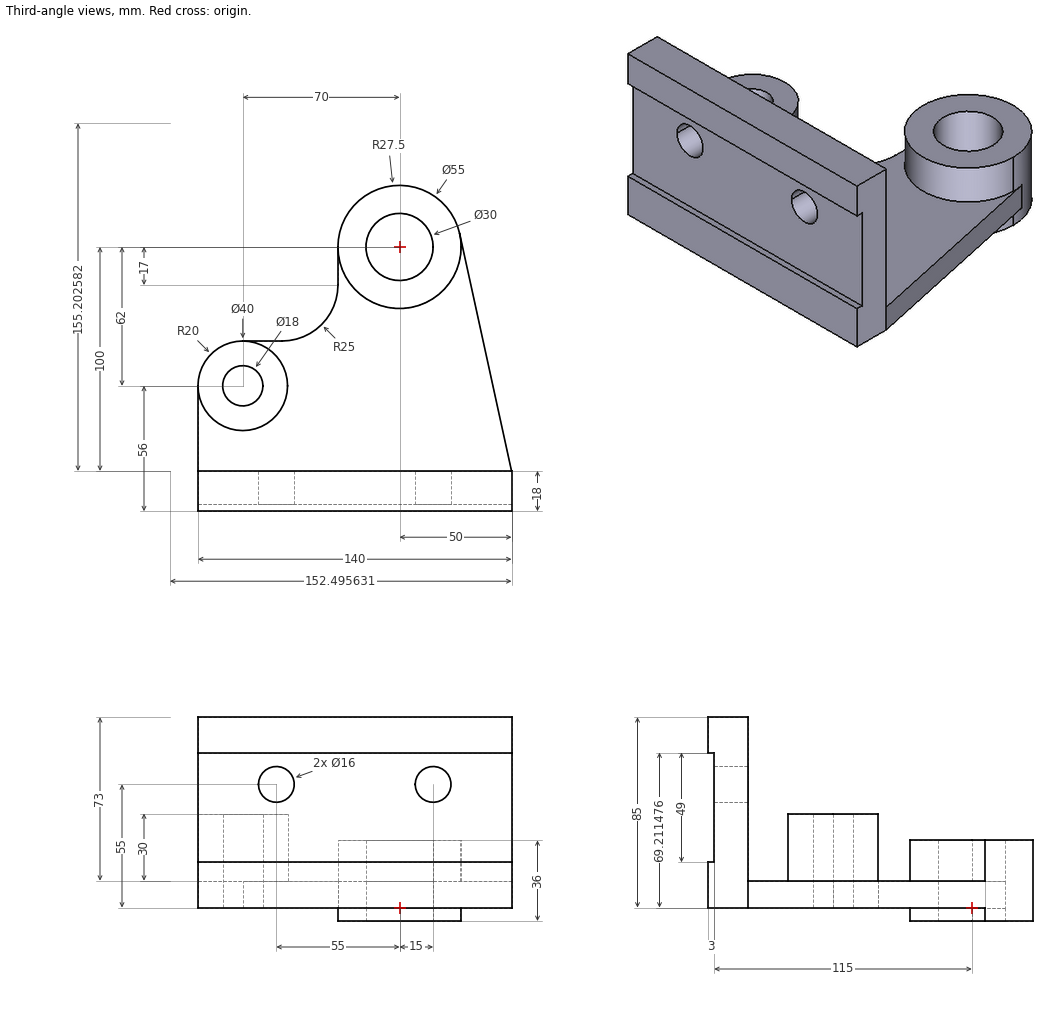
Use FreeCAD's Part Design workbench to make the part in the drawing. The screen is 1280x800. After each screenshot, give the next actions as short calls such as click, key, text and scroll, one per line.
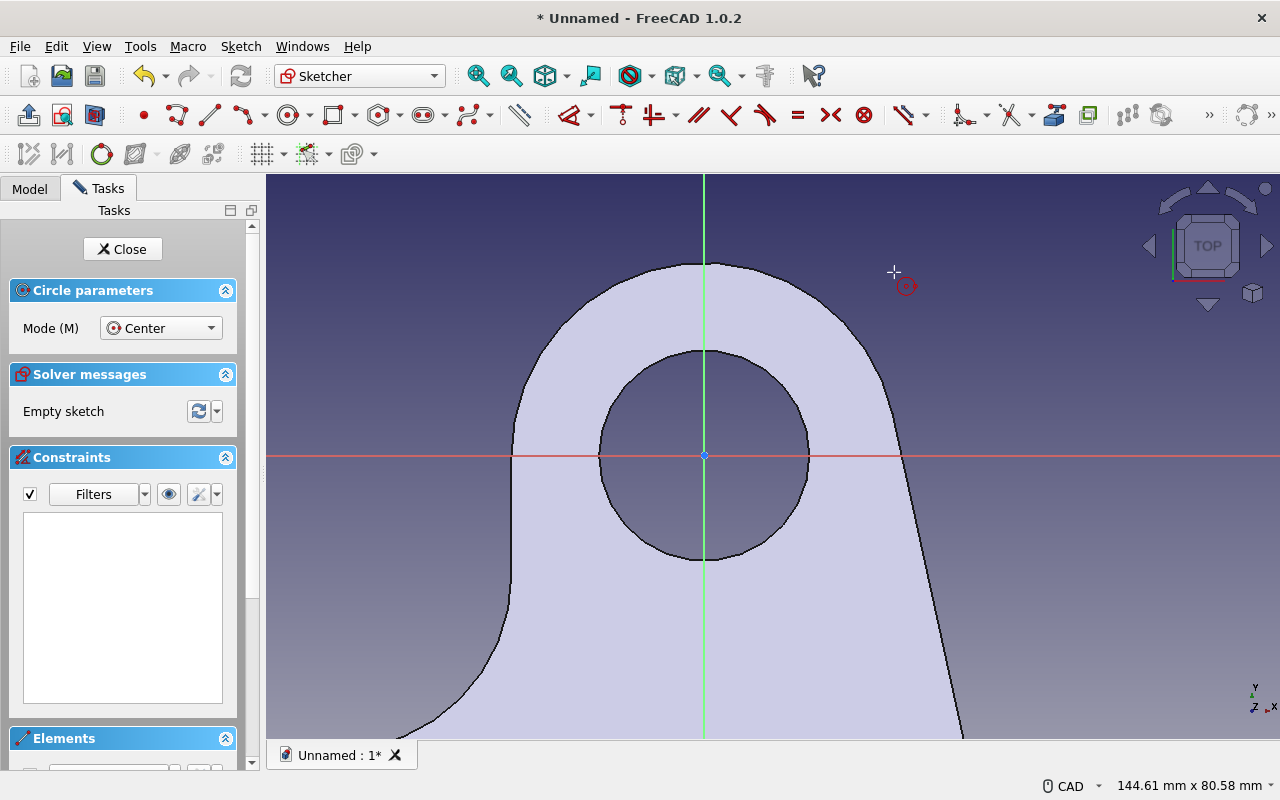
click(704, 456)
click(841, 319)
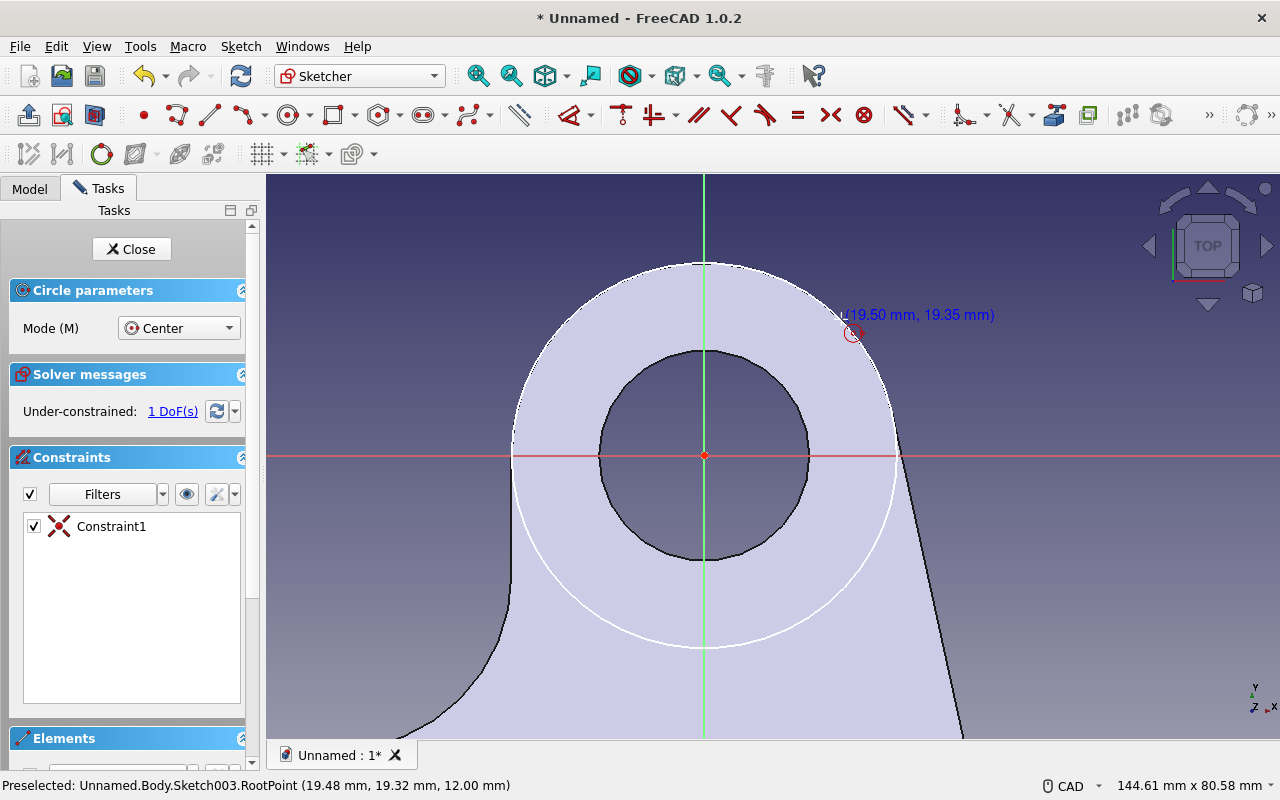
click(704, 456)
click(779, 381)
key(Escape)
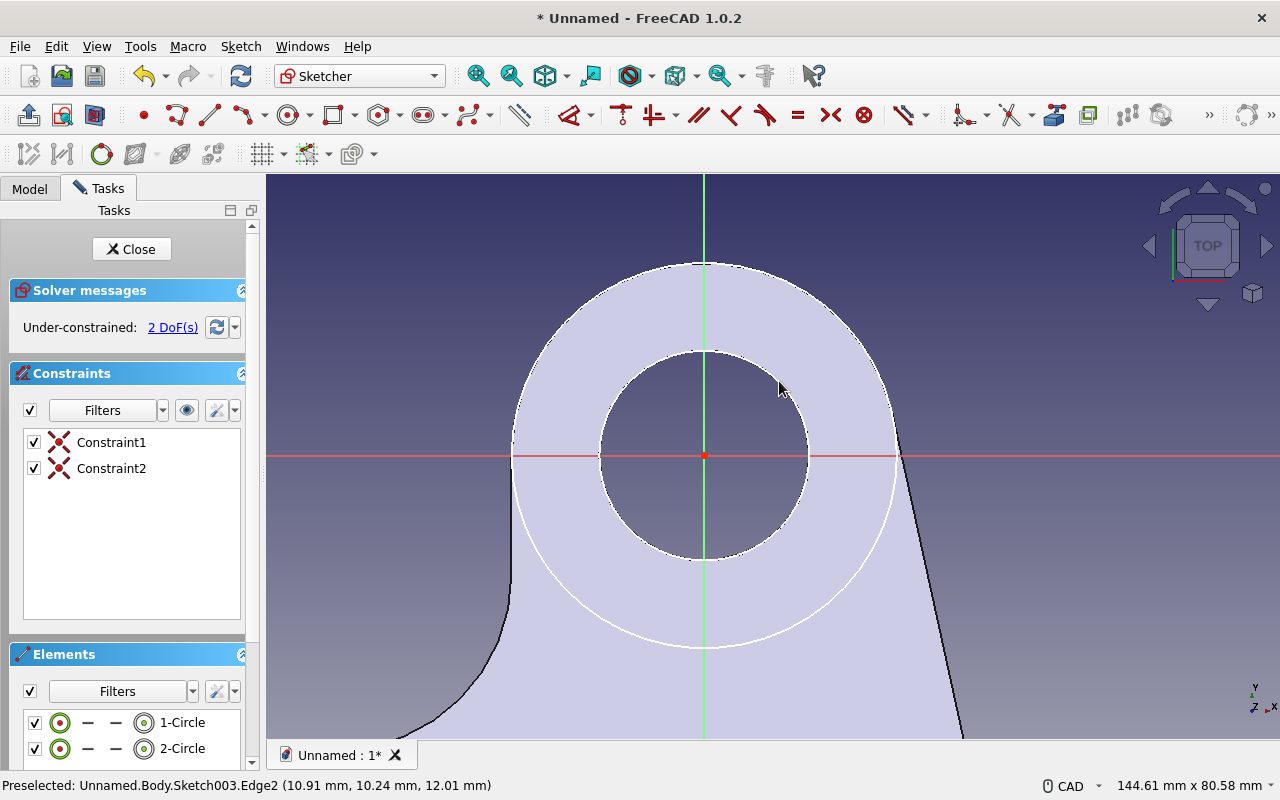
click(568, 116)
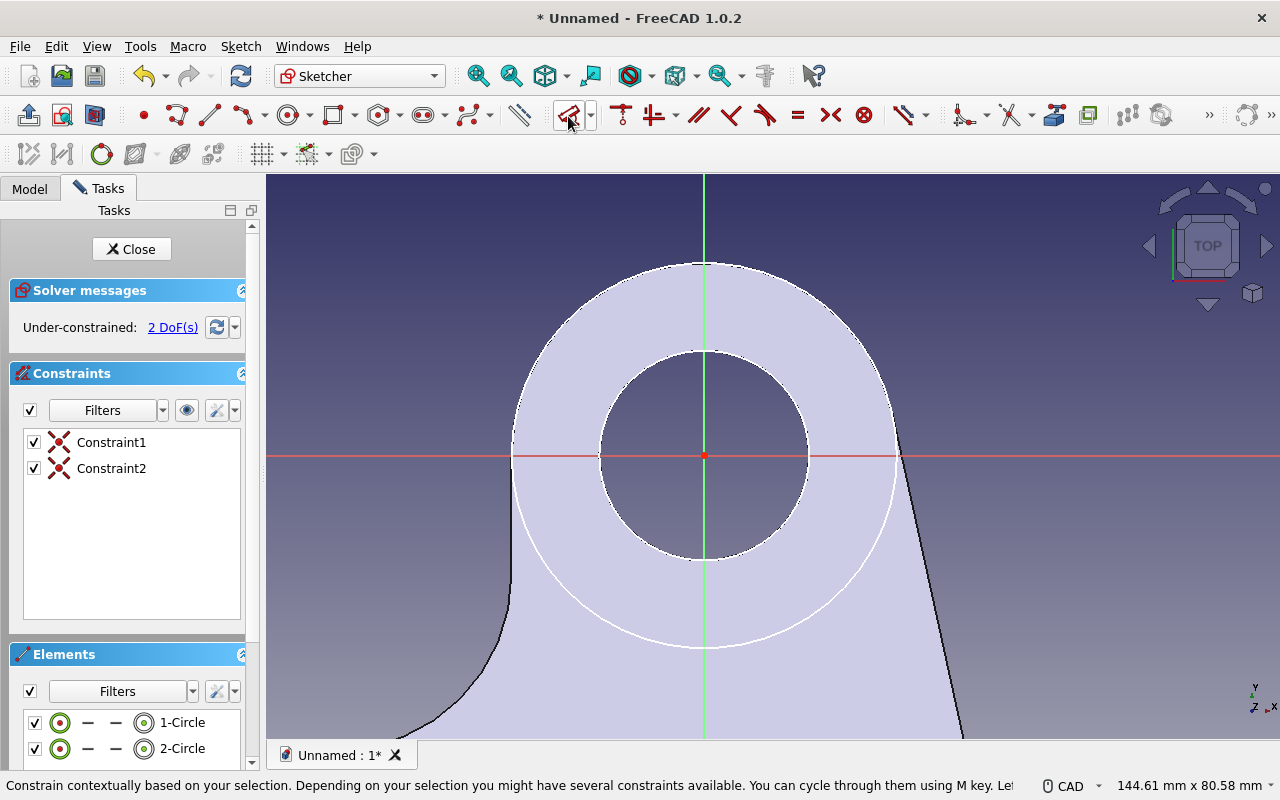
click(840, 319)
click(863, 296)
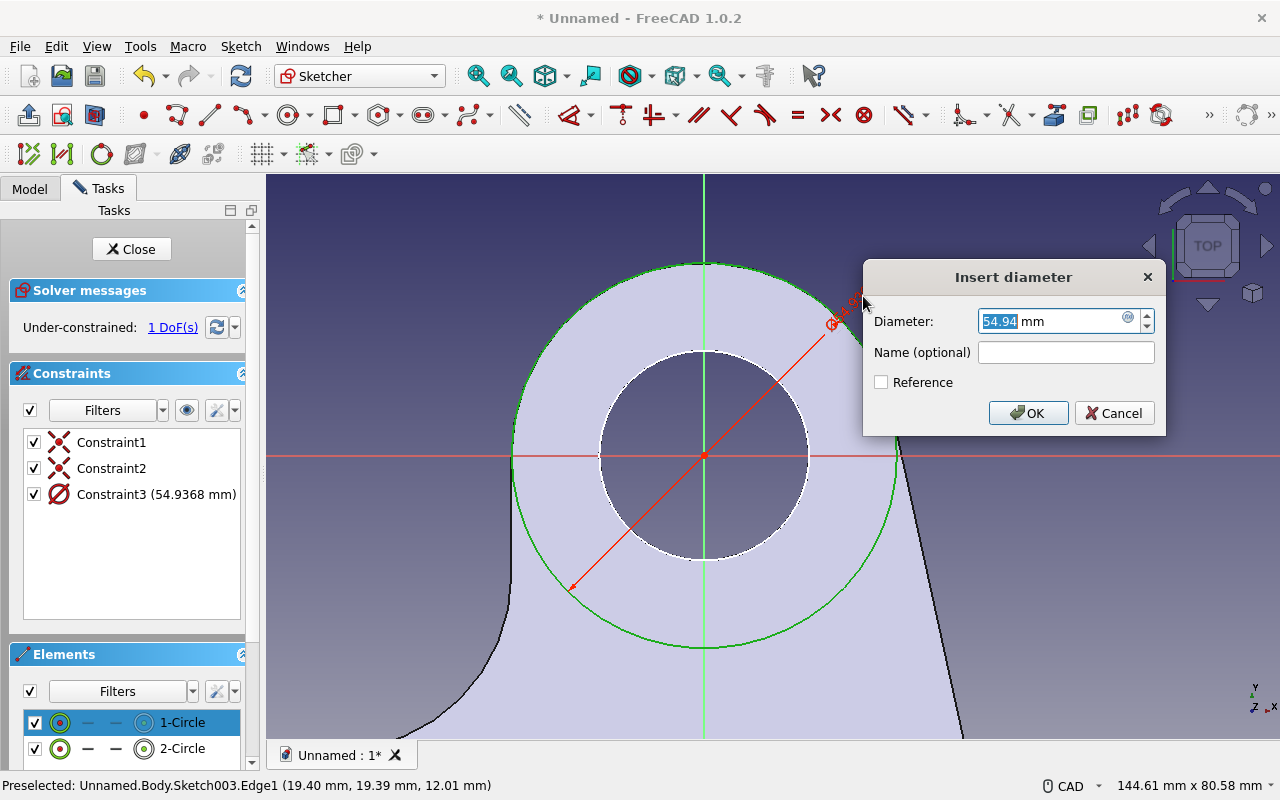
text(55)
key(Return)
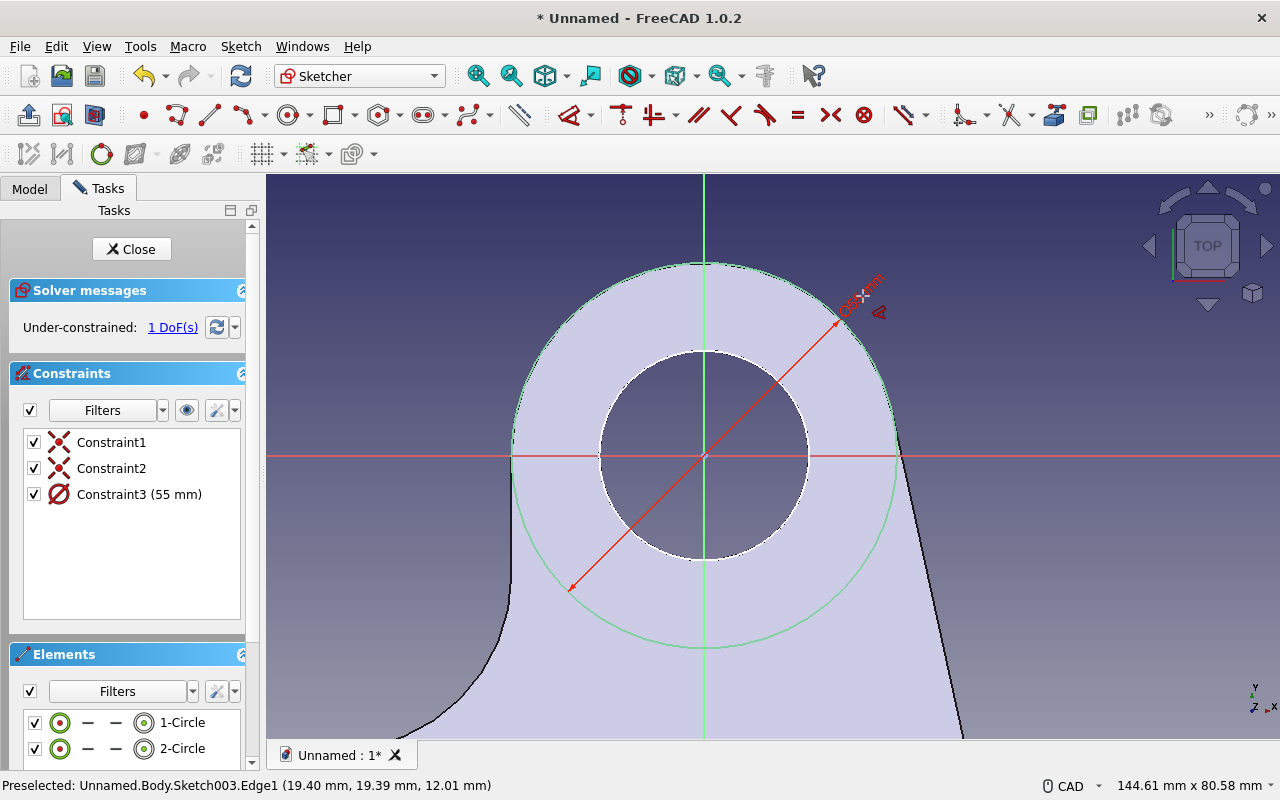
click(778, 381)
click(800, 358)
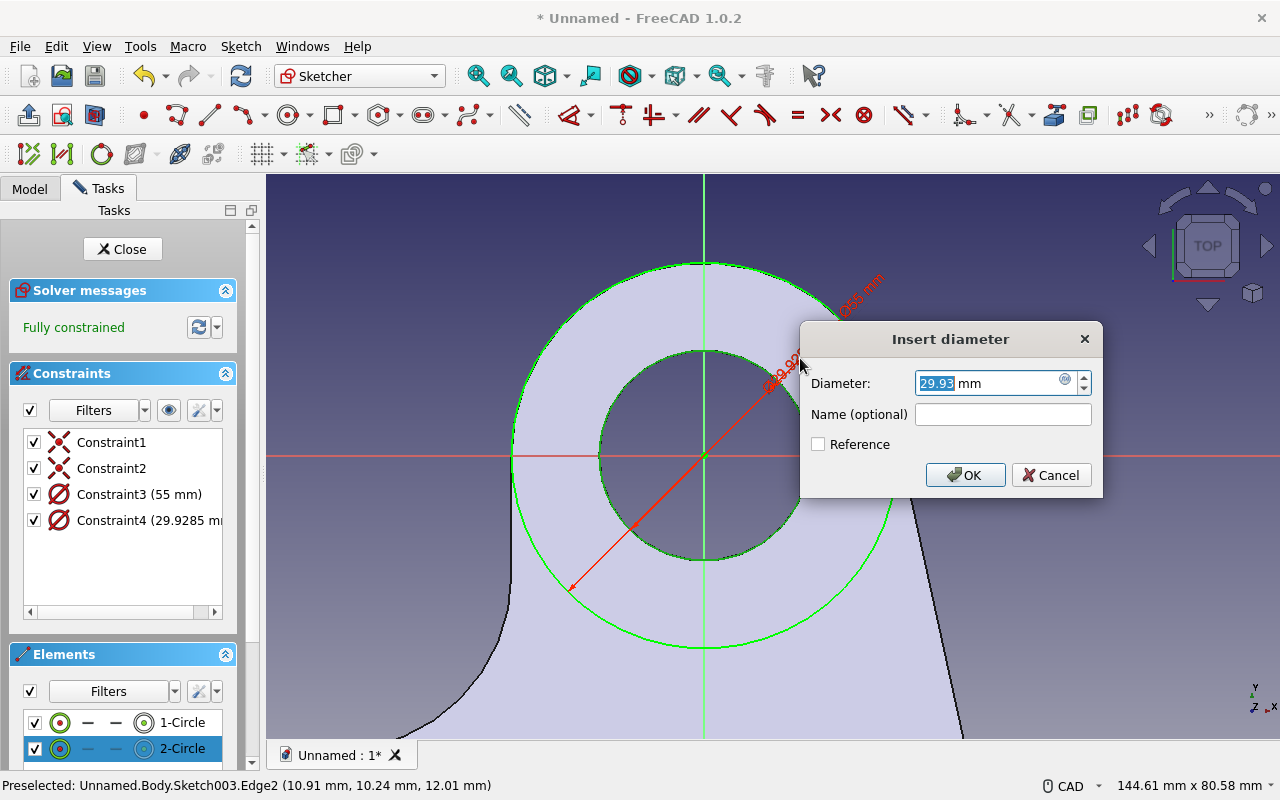
text(30)
key(Return)
key(Escape)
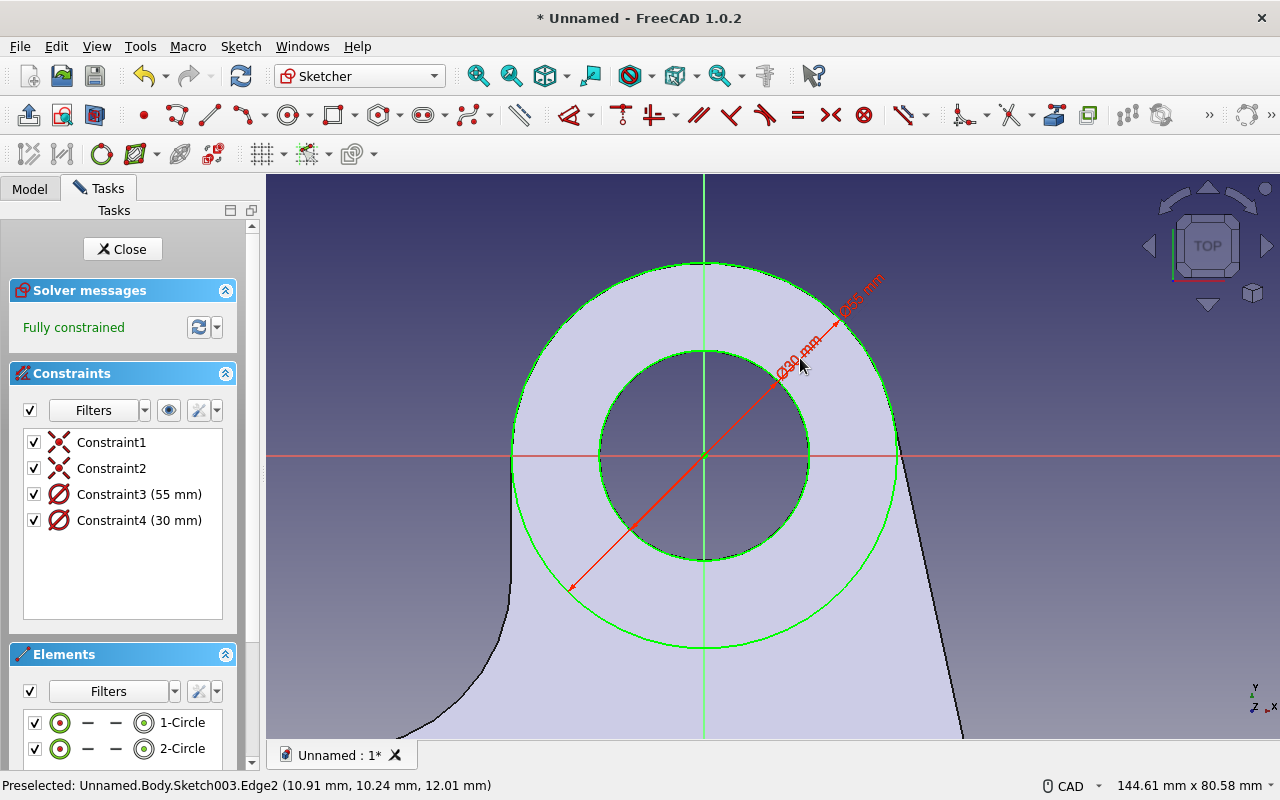
click(123, 249)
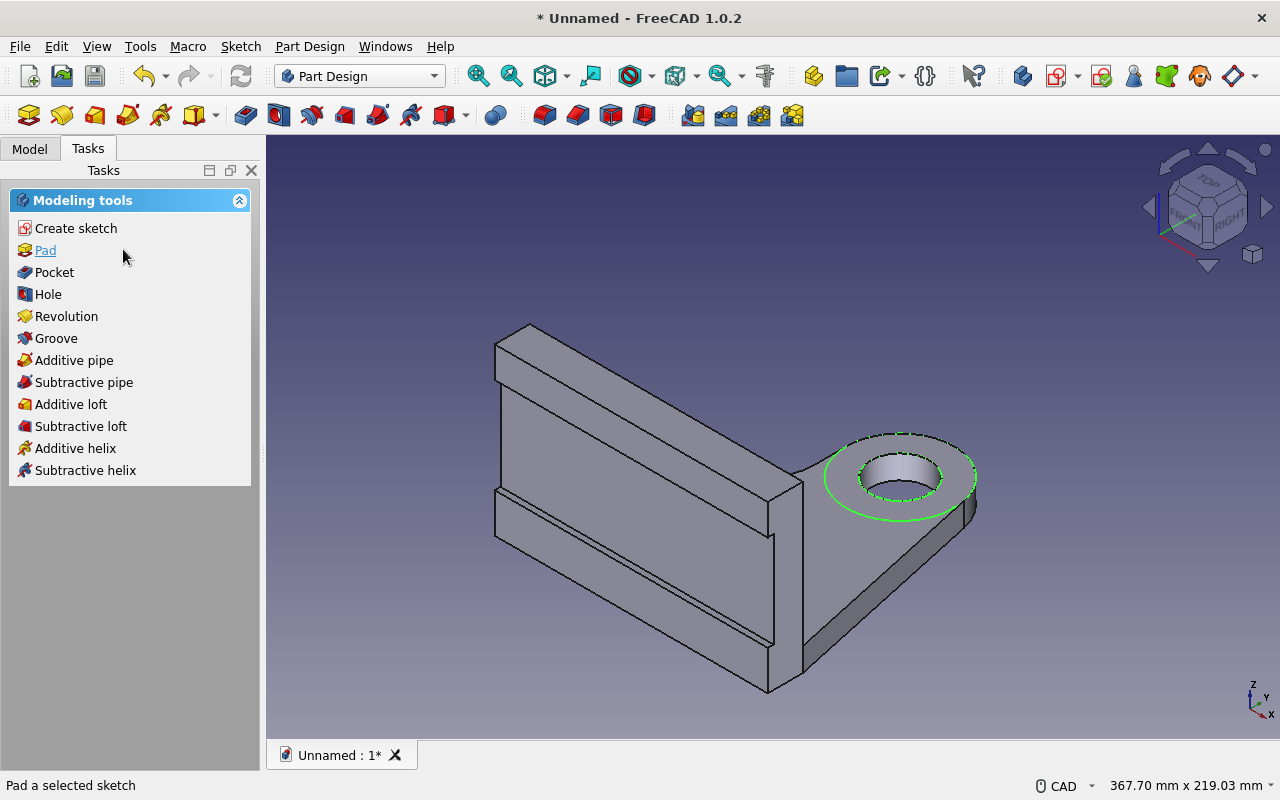
click(29, 116)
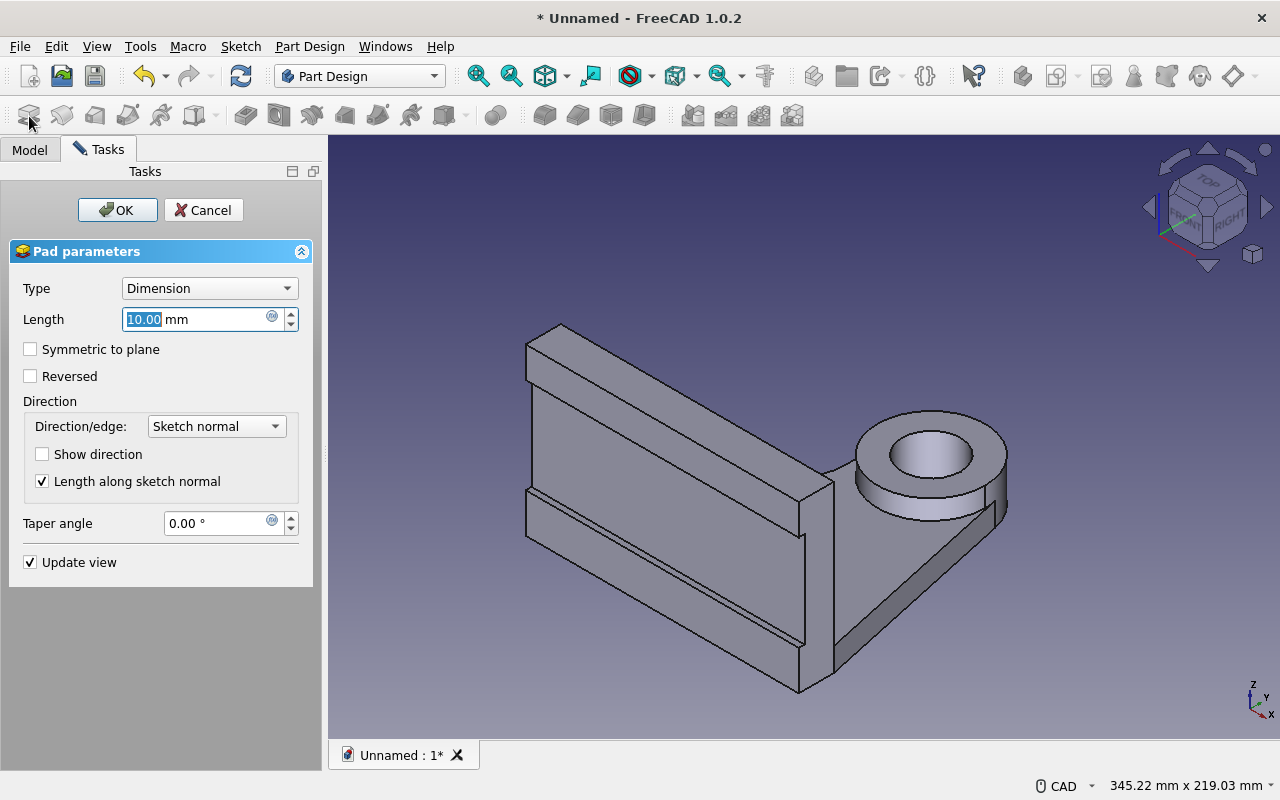
text(36)
key(Tab)